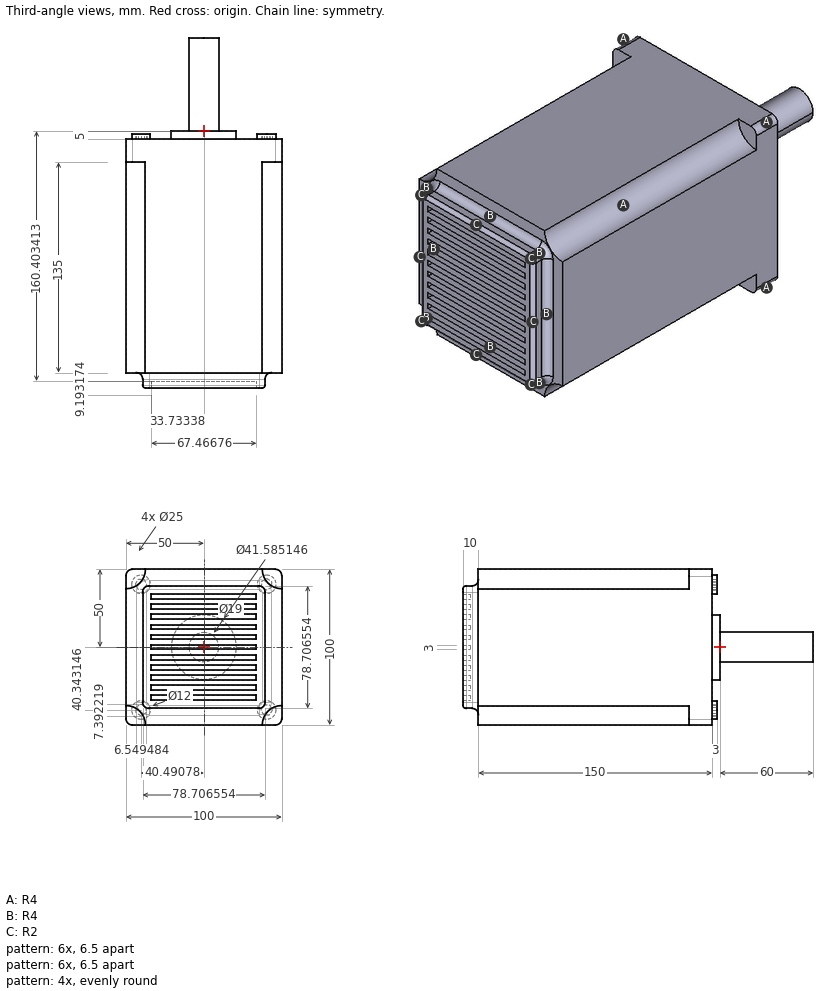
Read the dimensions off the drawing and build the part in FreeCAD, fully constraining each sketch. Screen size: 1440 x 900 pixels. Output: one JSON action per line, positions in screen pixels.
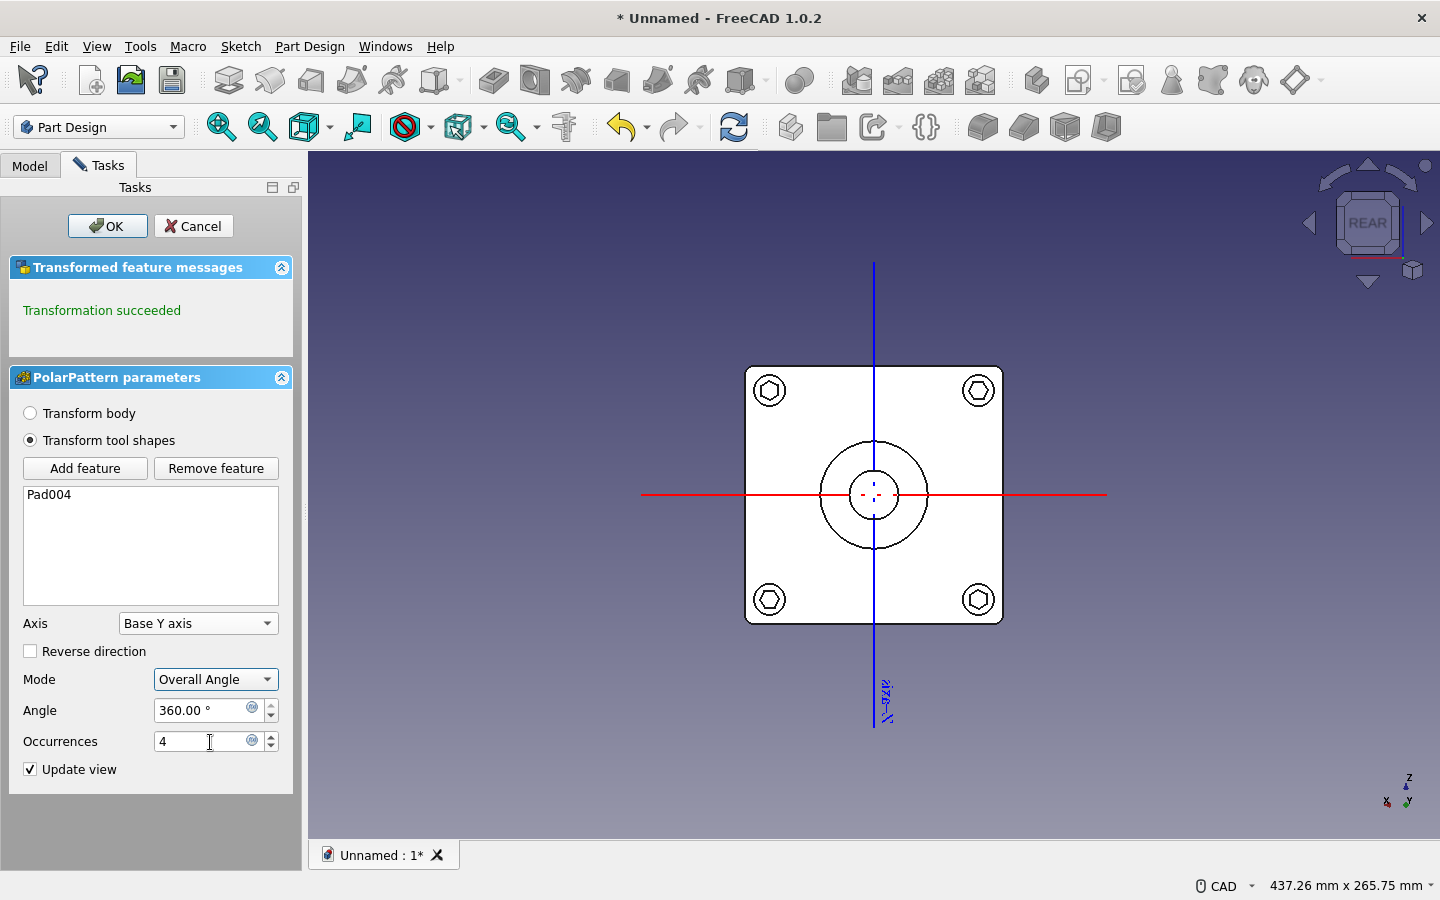
{"action": "left_click", "coordinate": [108, 226]}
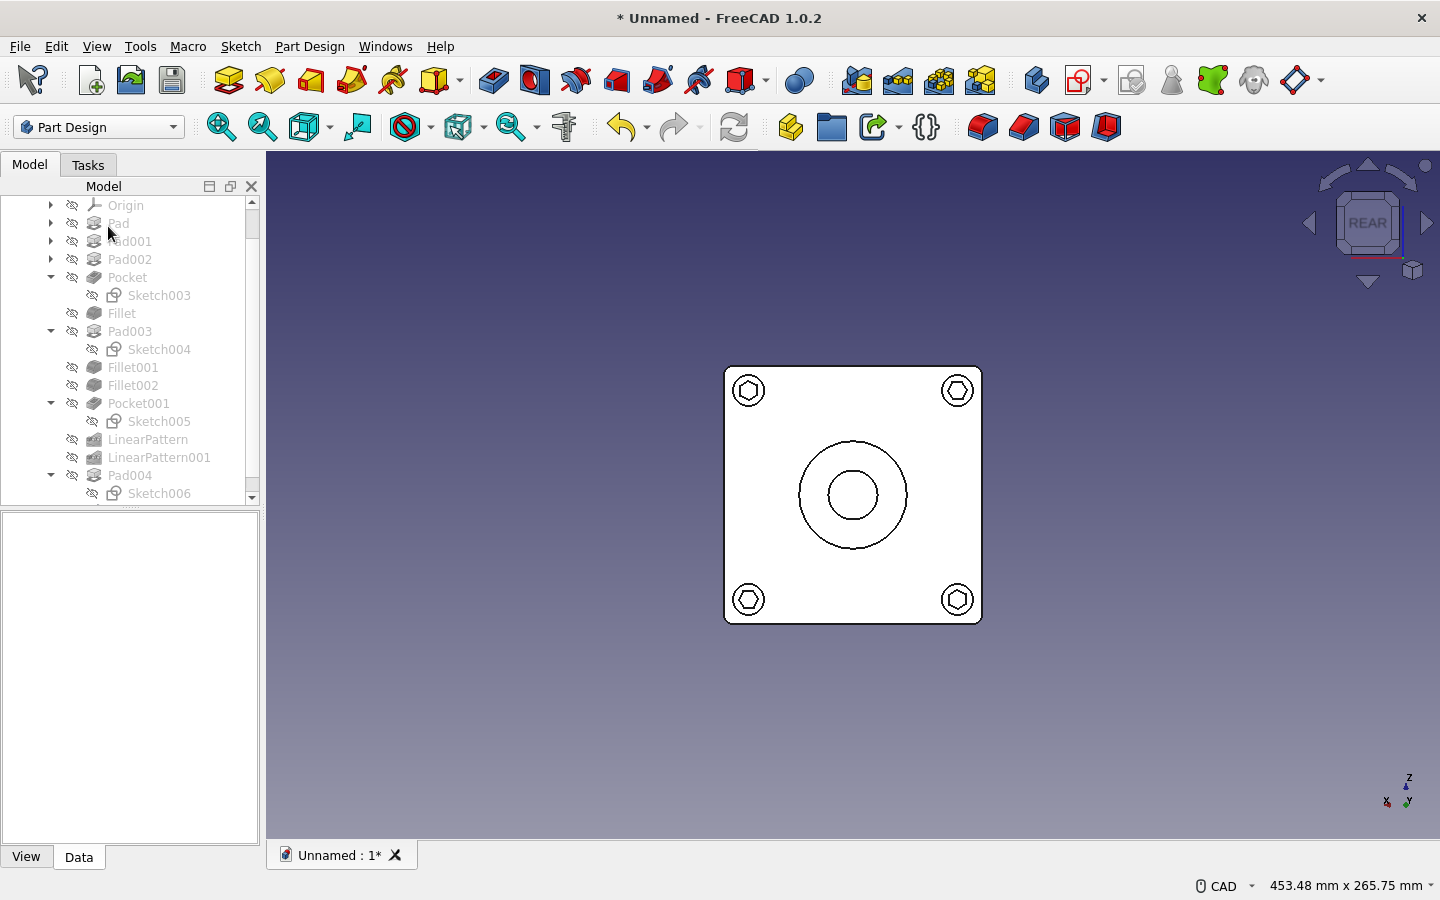
{"action": "key", "text": "0"}